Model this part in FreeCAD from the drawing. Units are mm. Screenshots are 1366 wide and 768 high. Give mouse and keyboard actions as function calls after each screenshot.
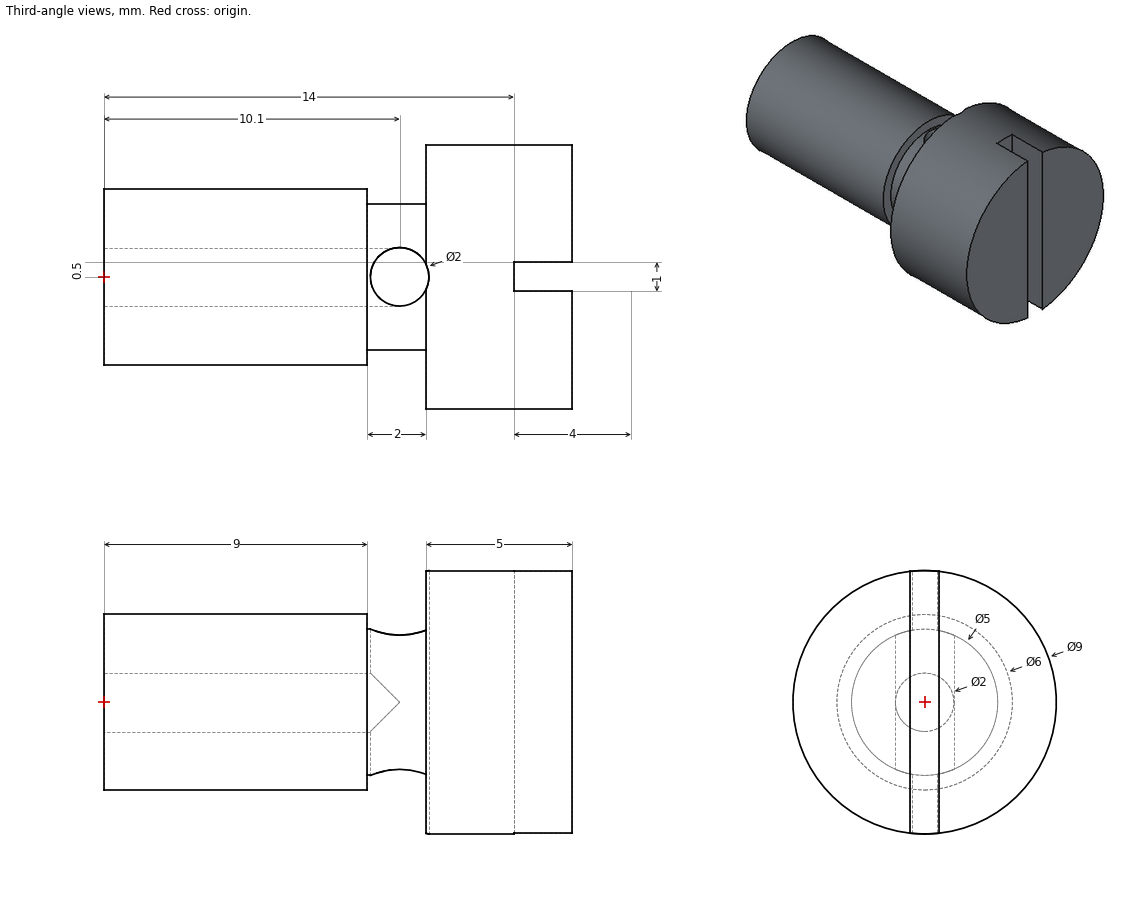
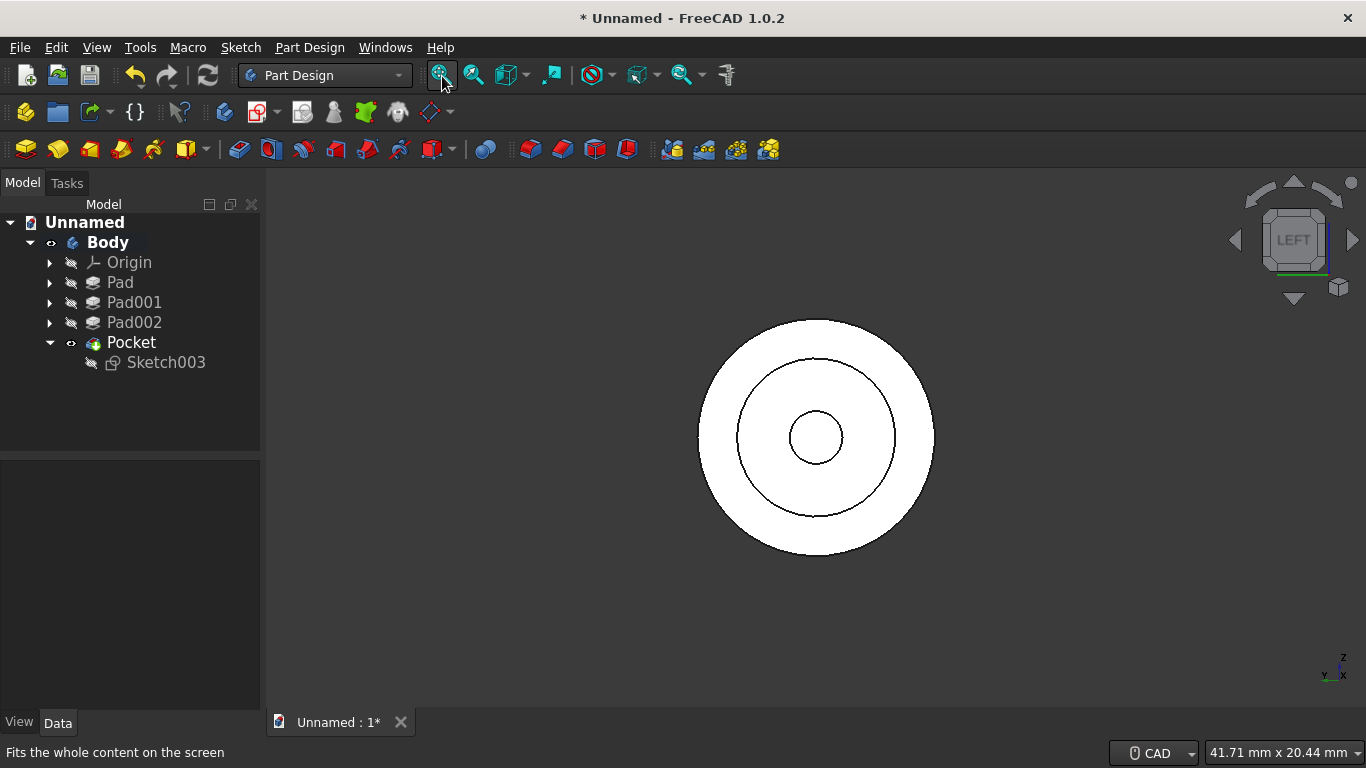
click(258, 112)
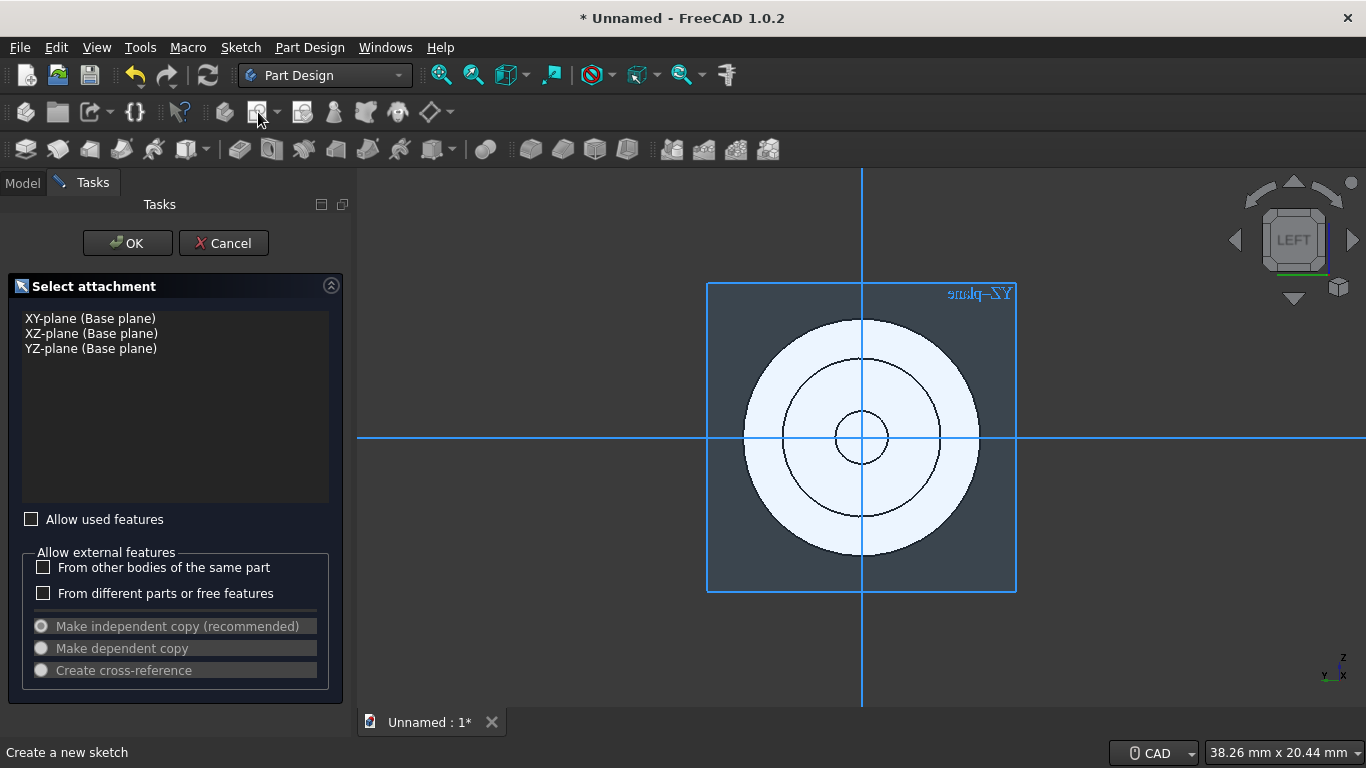
click(82, 318)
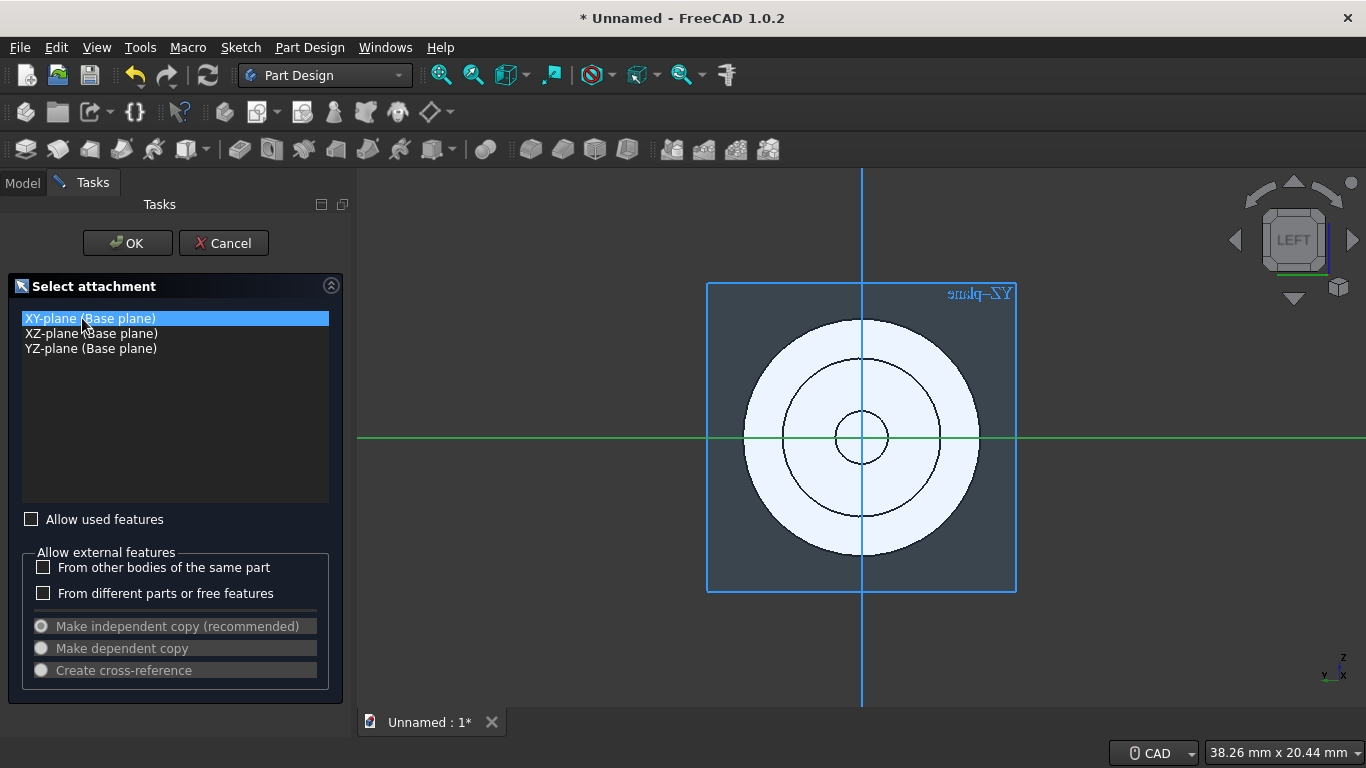
click(128, 243)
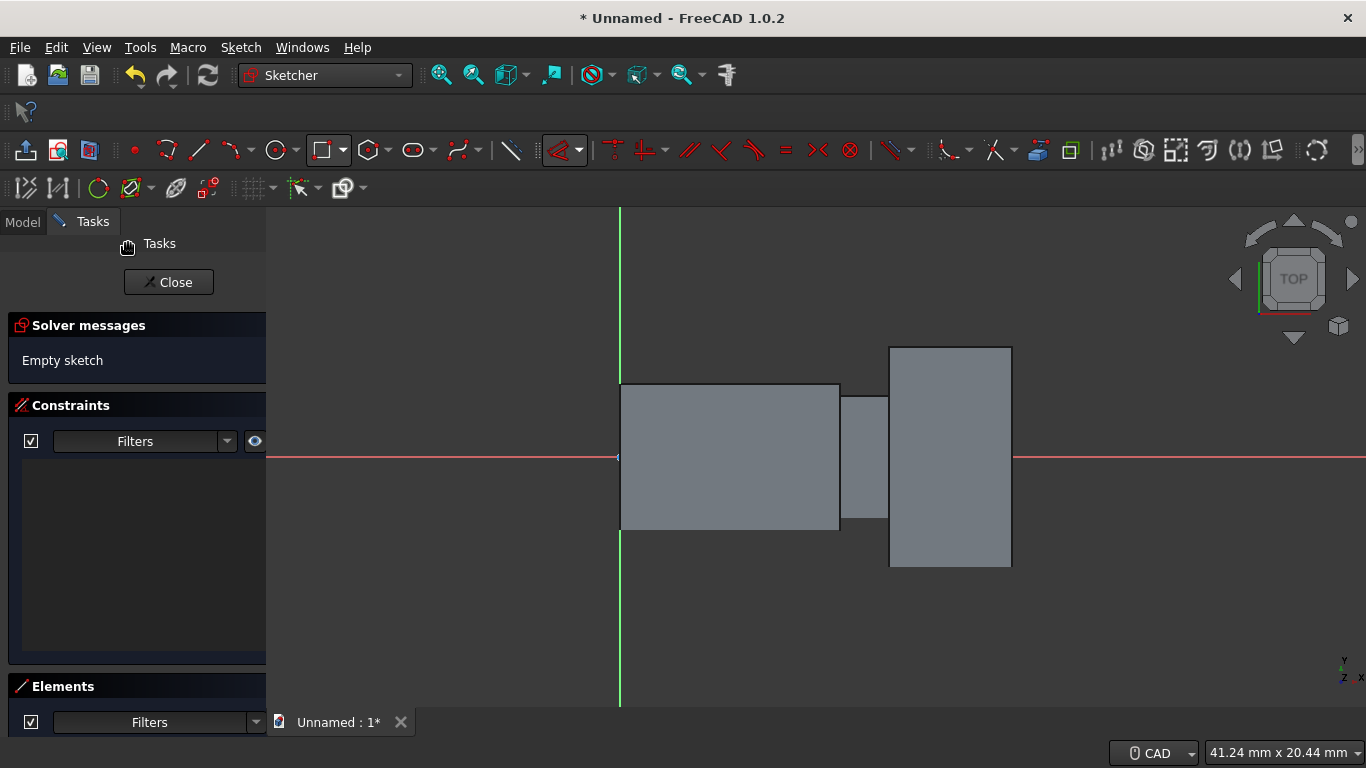
click(90, 150)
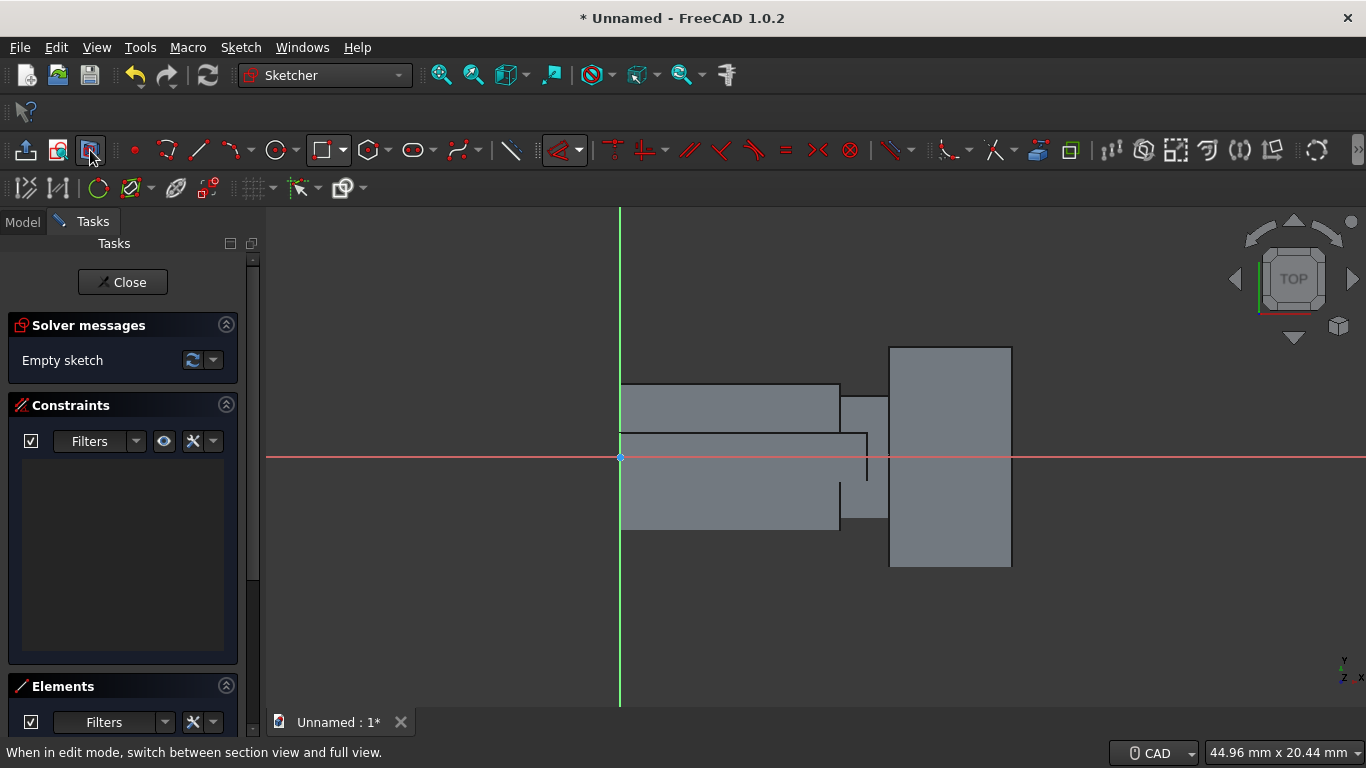
scroll(891, 457, up, 9)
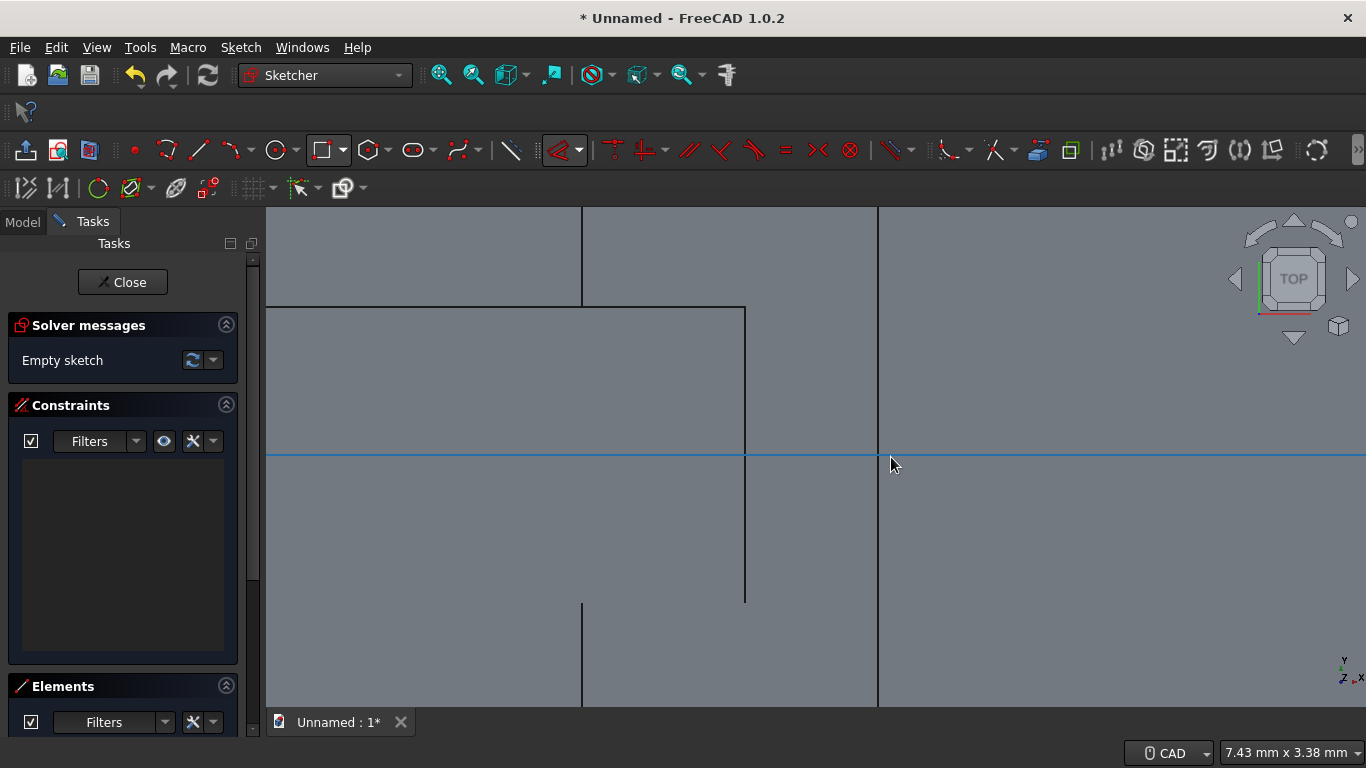
click(276, 150)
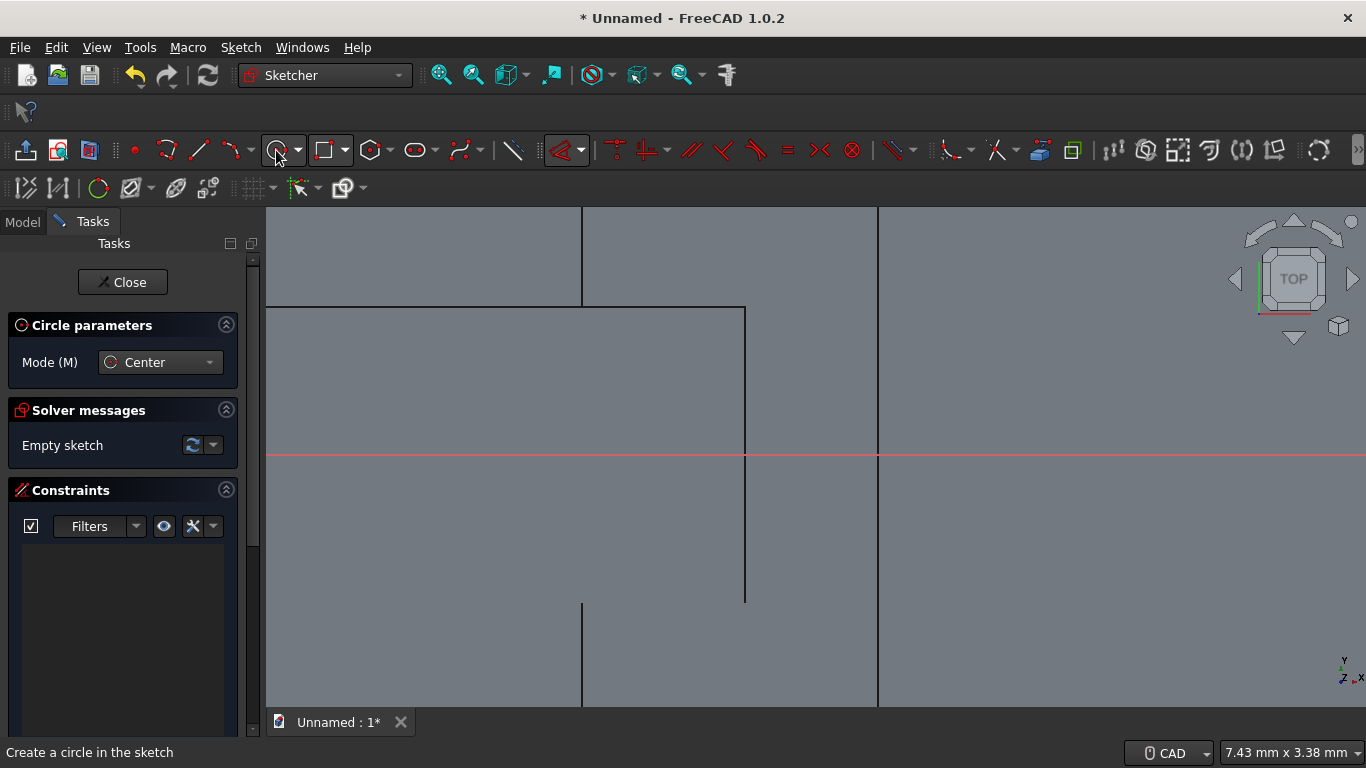
click(745, 455)
click(850, 351)
key(Escape)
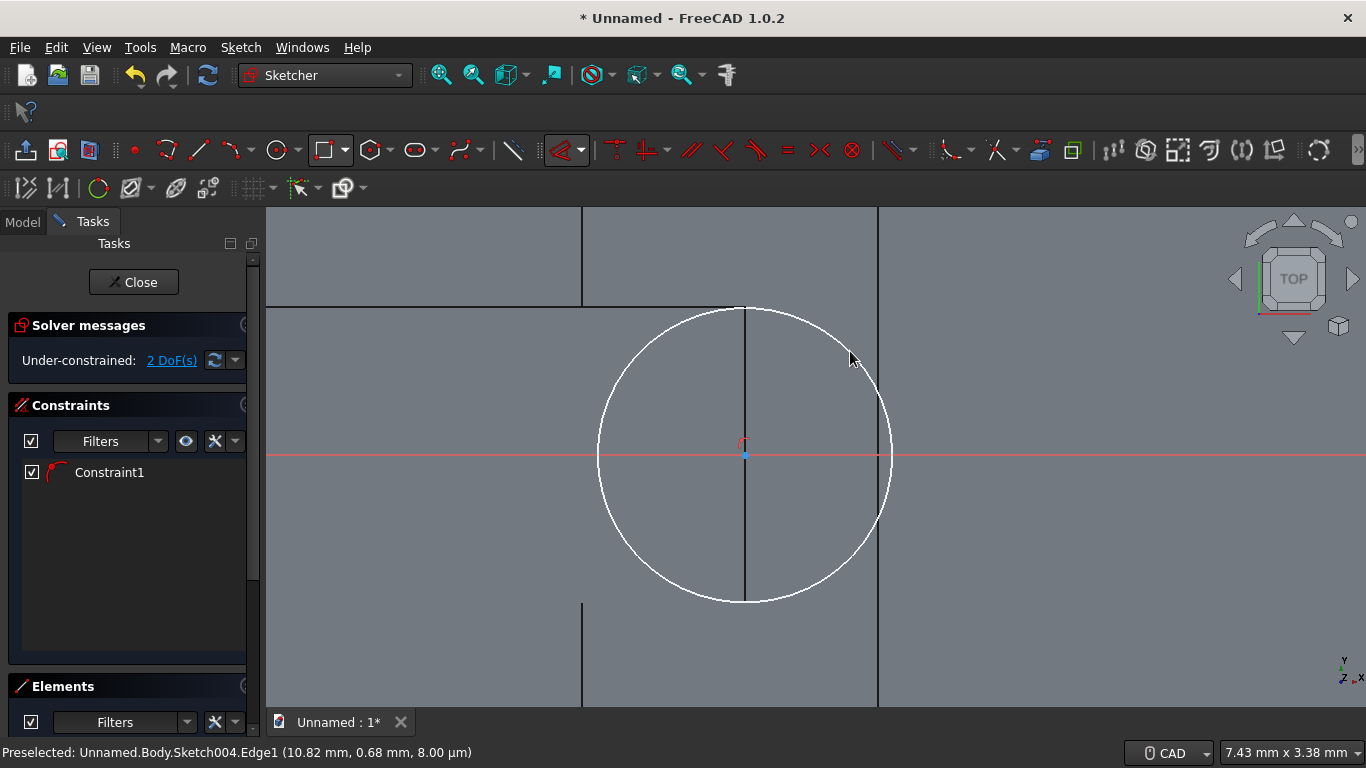
click(849, 351)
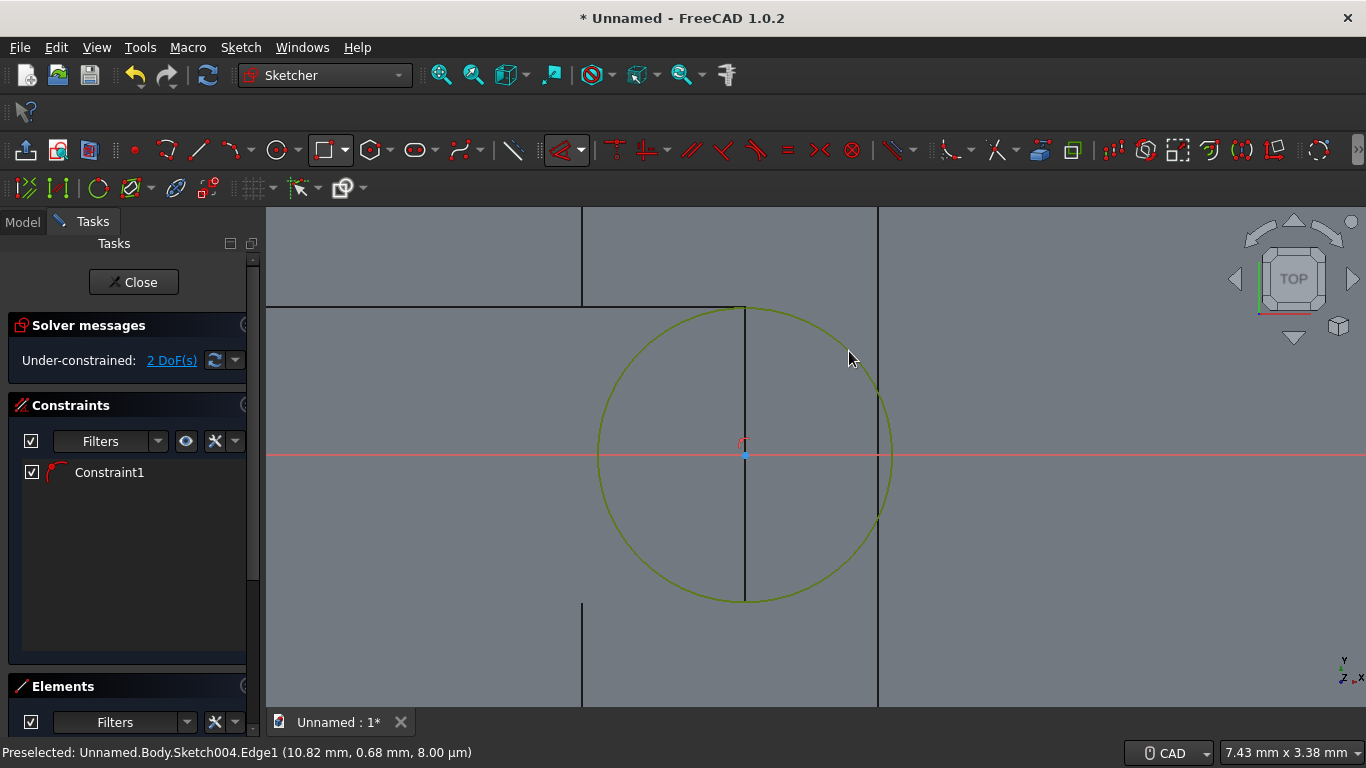
key(k)
key(o)